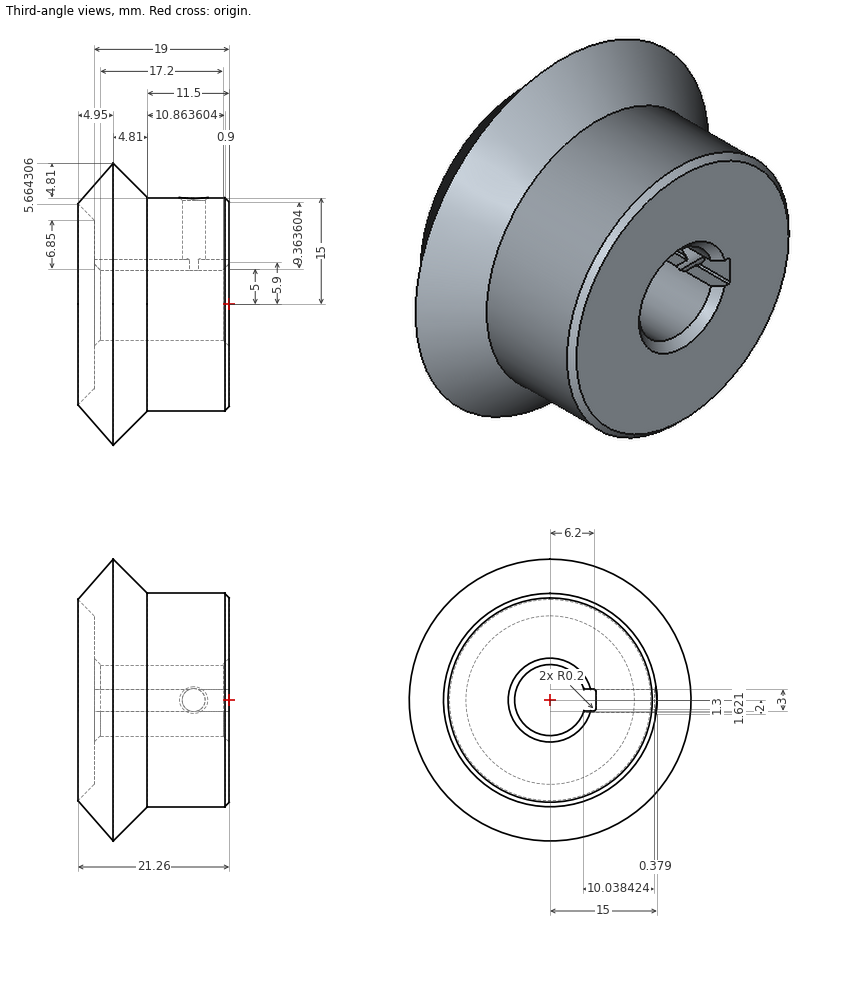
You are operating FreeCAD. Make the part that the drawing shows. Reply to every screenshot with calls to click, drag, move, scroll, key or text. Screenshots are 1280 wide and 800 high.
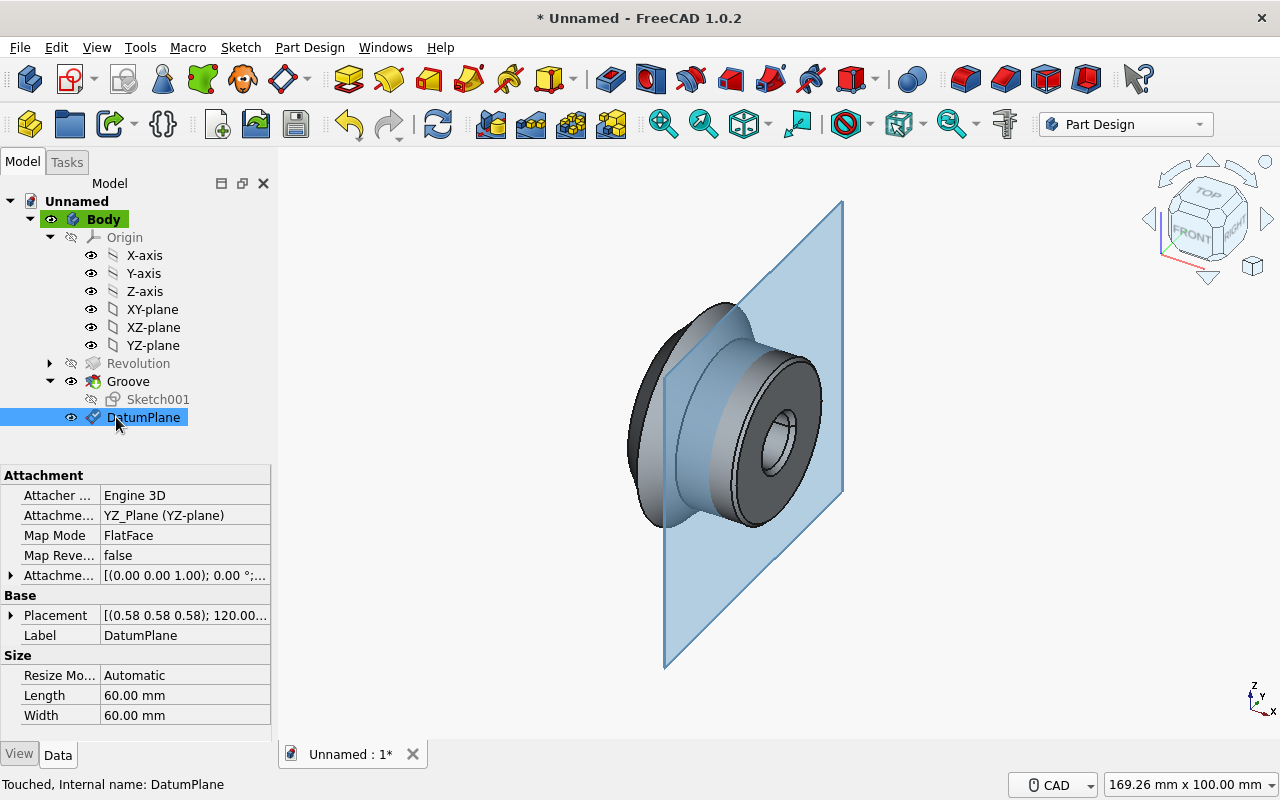
click(70, 80)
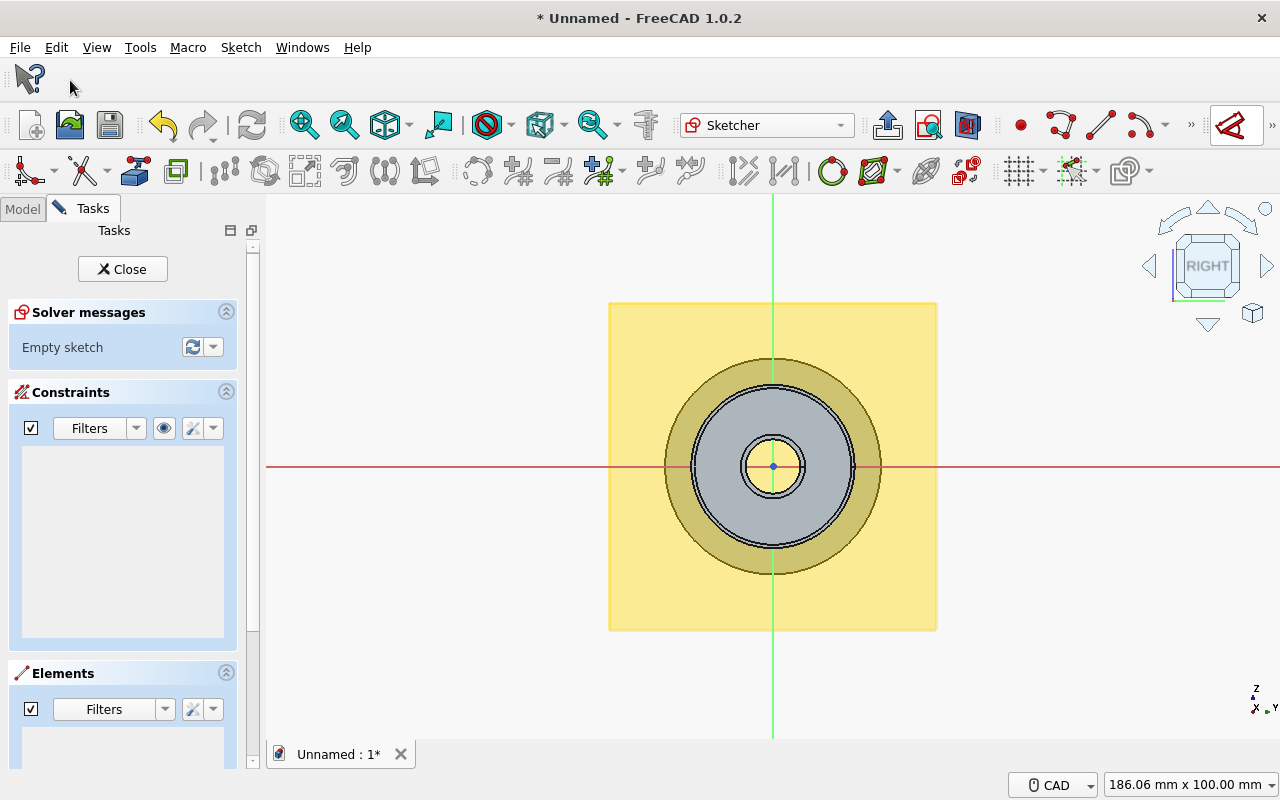
click(968, 126)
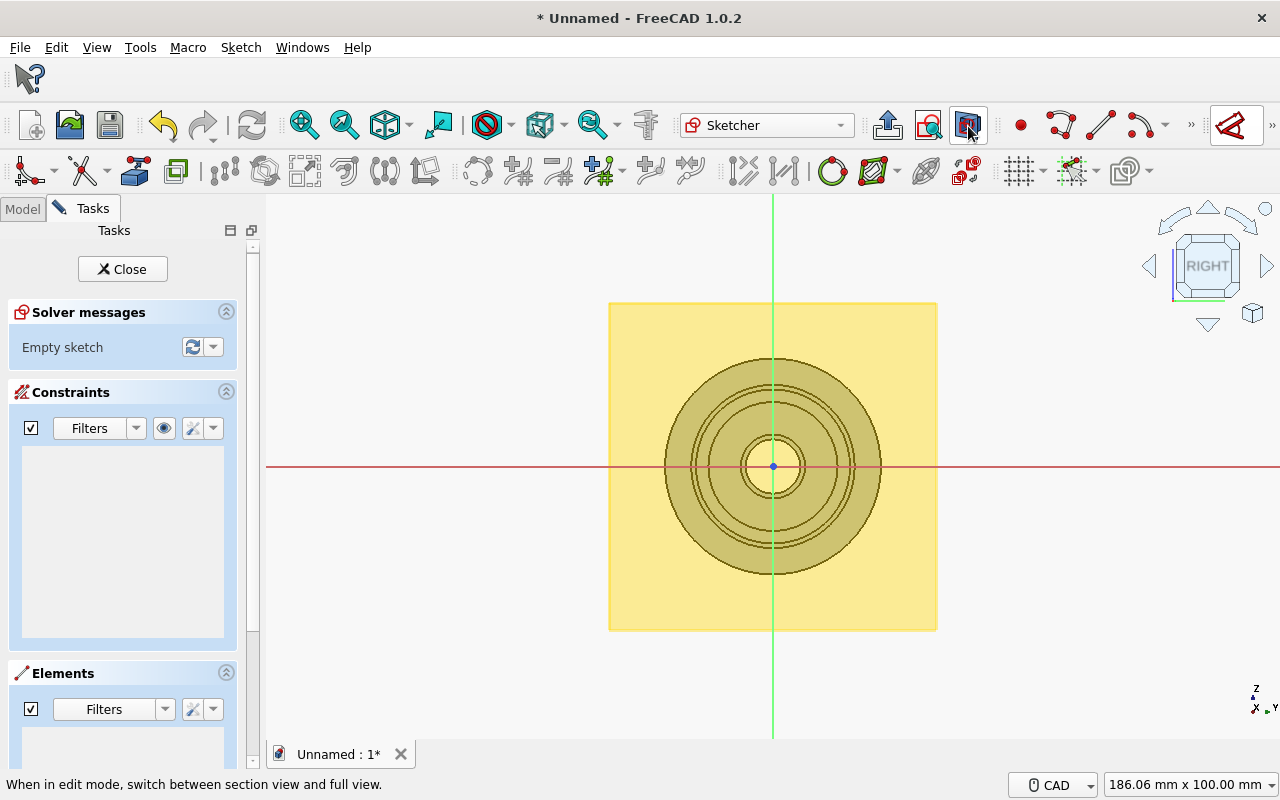
scroll(831, 473, up, 10)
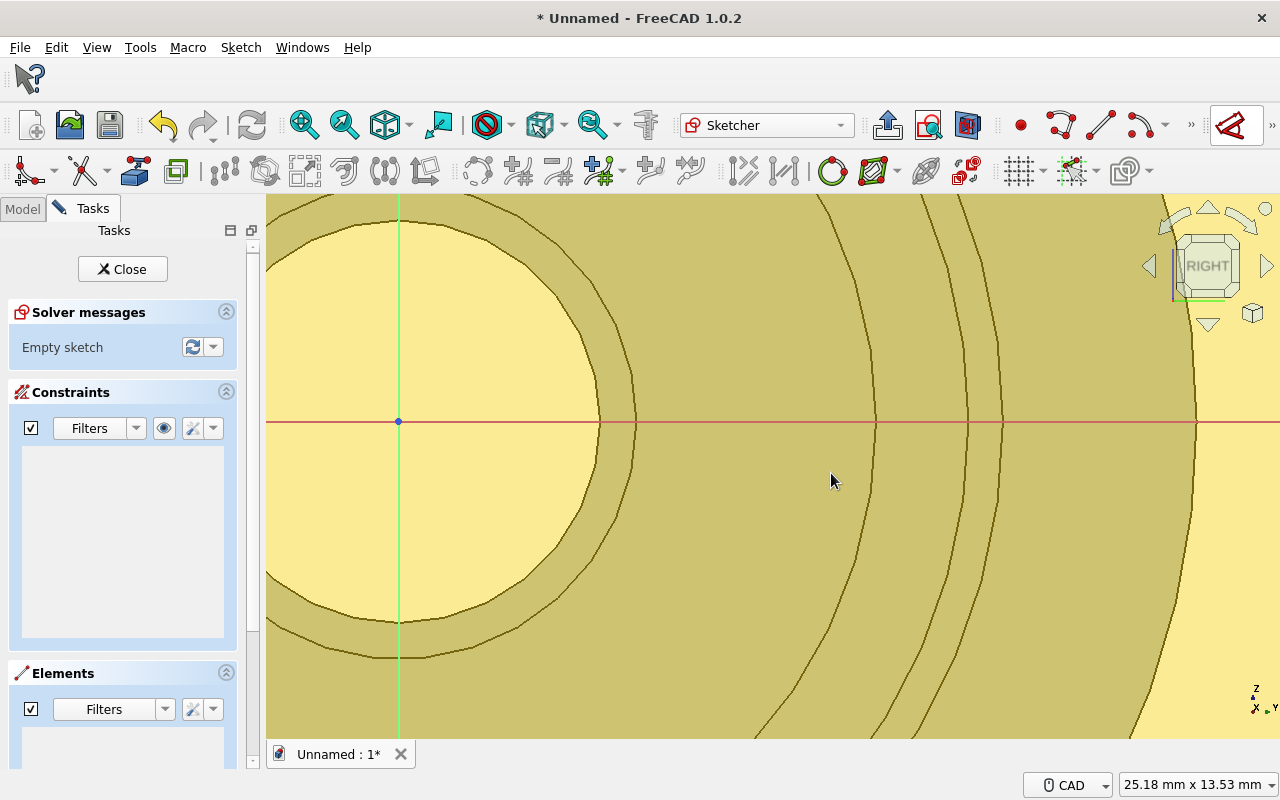
click(1062, 126)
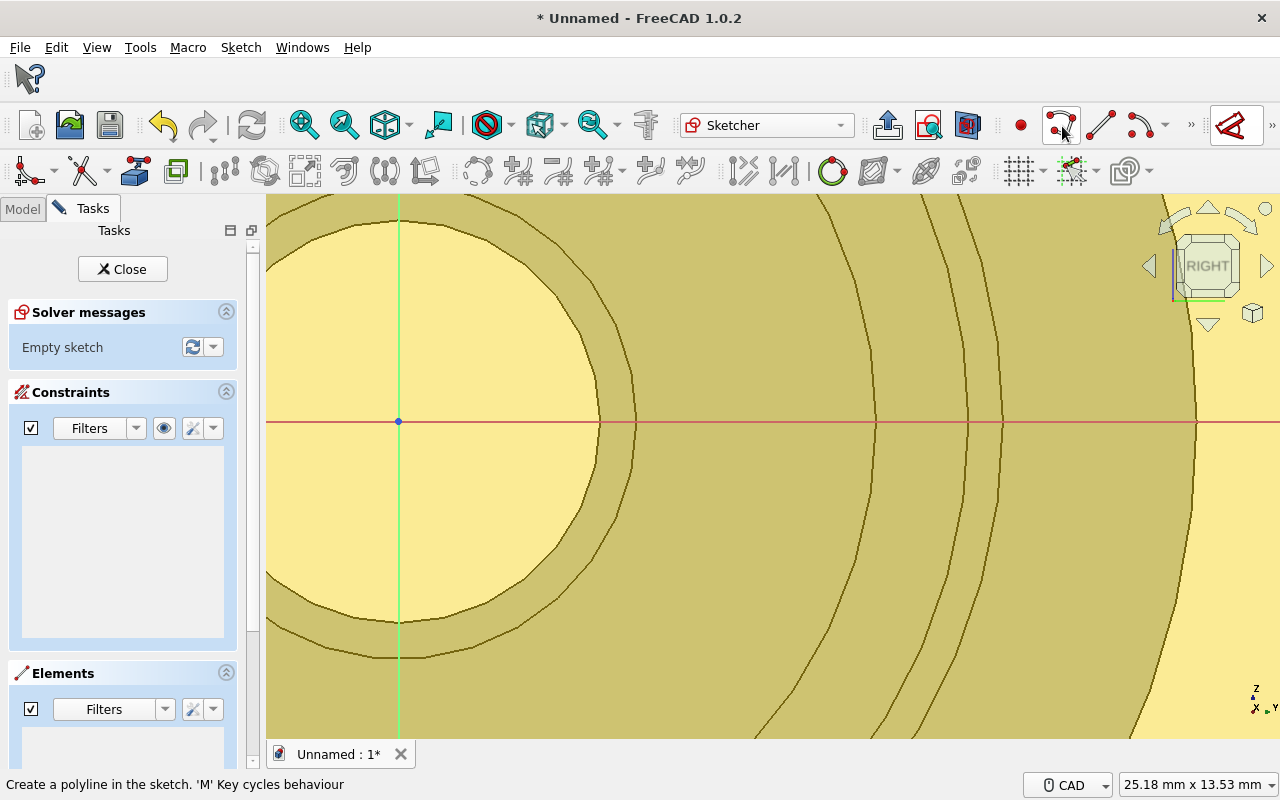
click(583, 422)
click(583, 487)
click(988, 487)
click(1003, 502)
click(1003, 431)
click(583, 422)
key(Escape)
key(Escape)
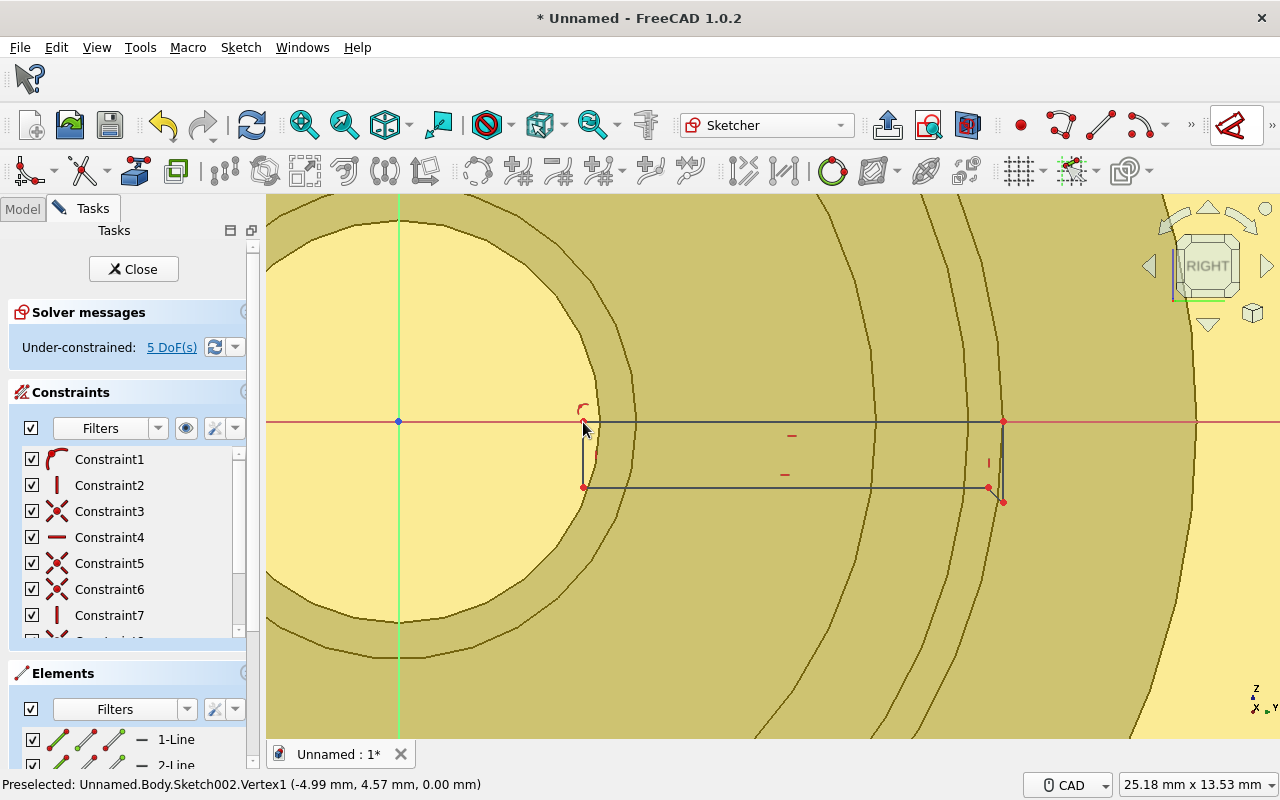
click(1003, 479)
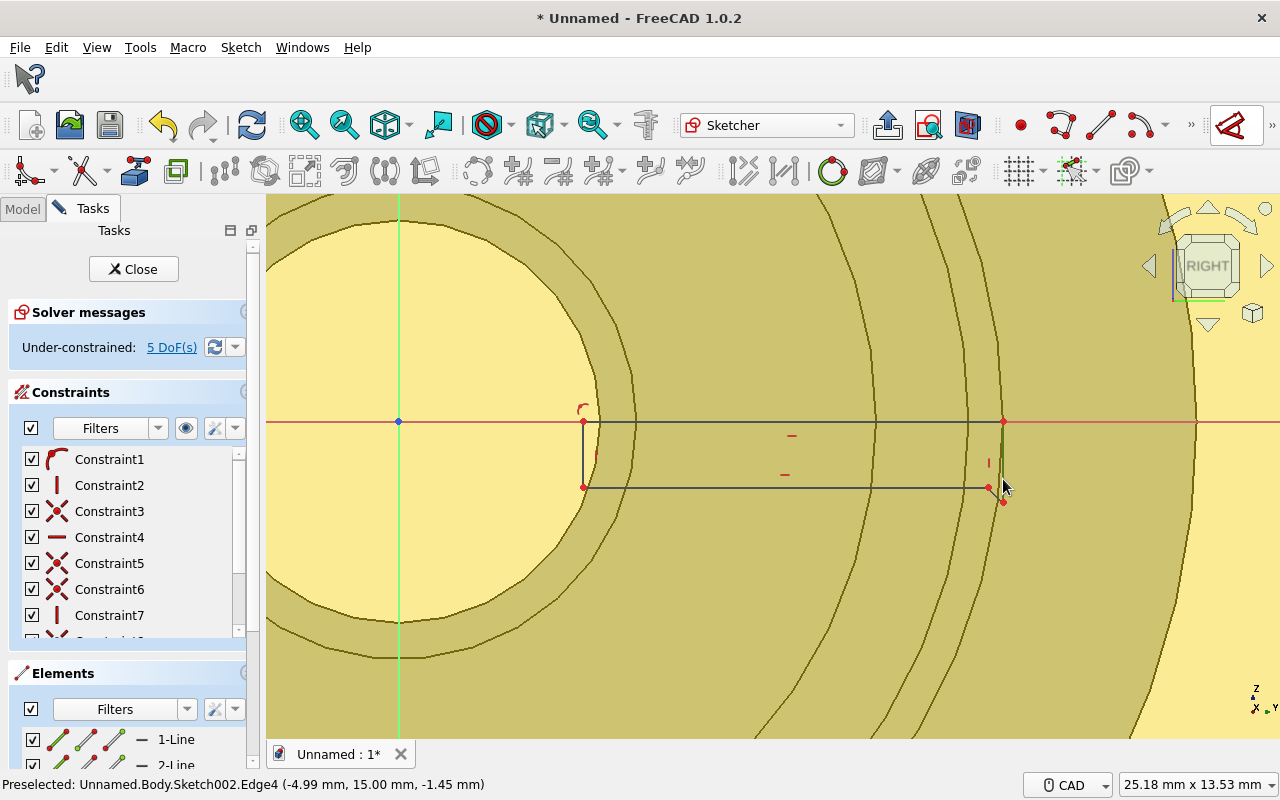
click(1258, 126)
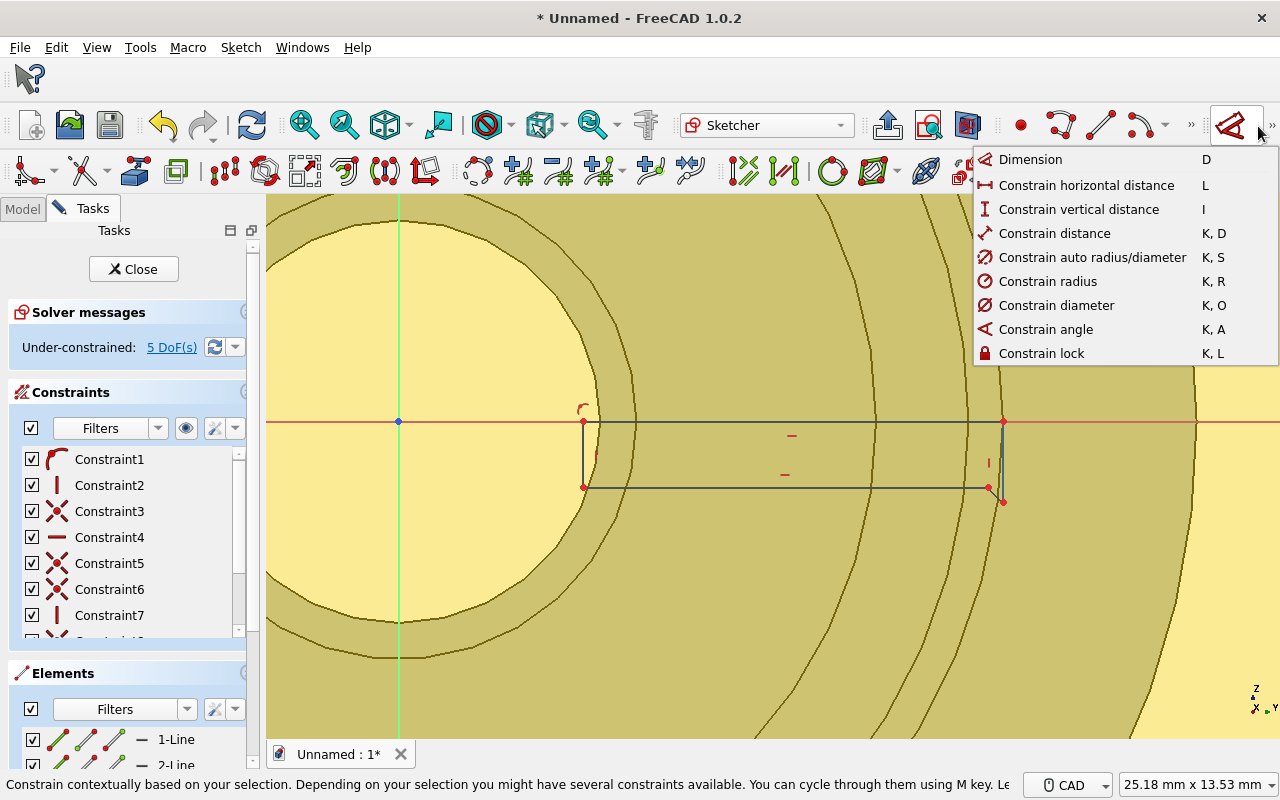
click(1126, 209)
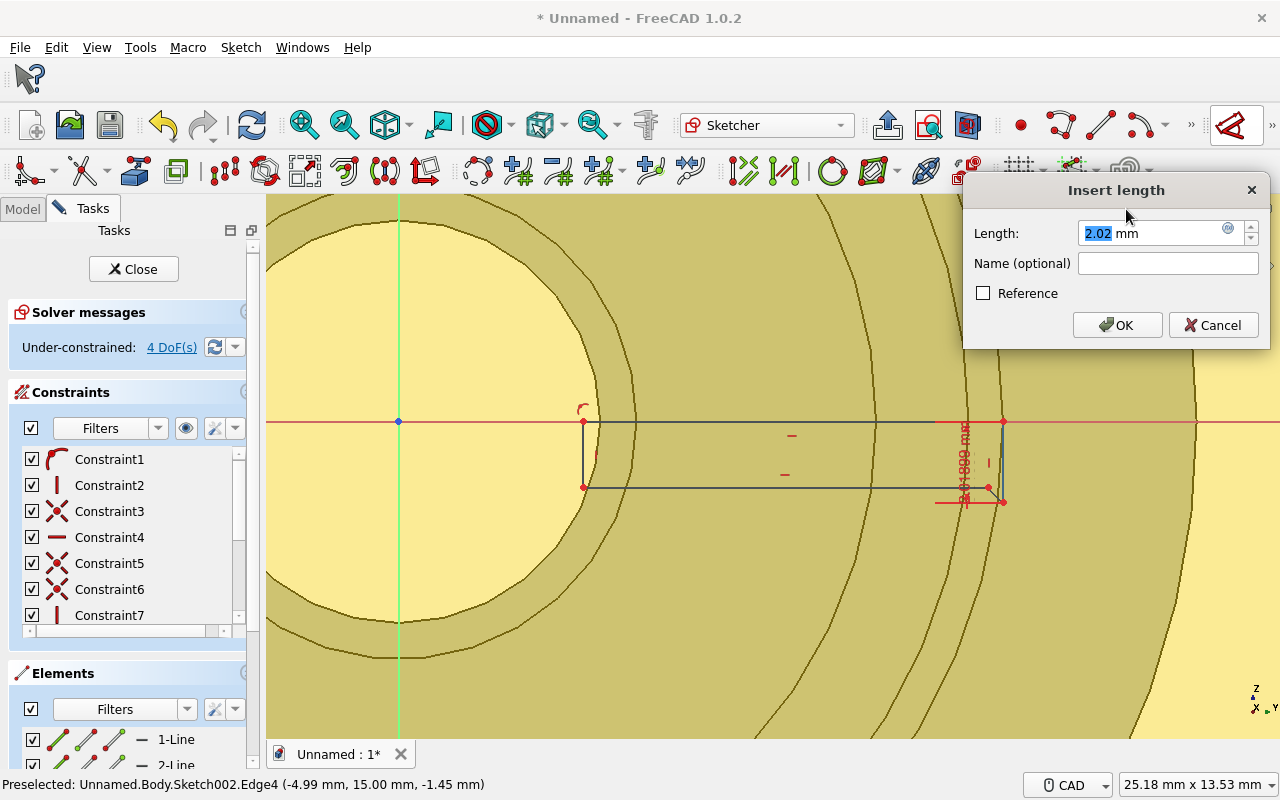
text(2)
key(Return)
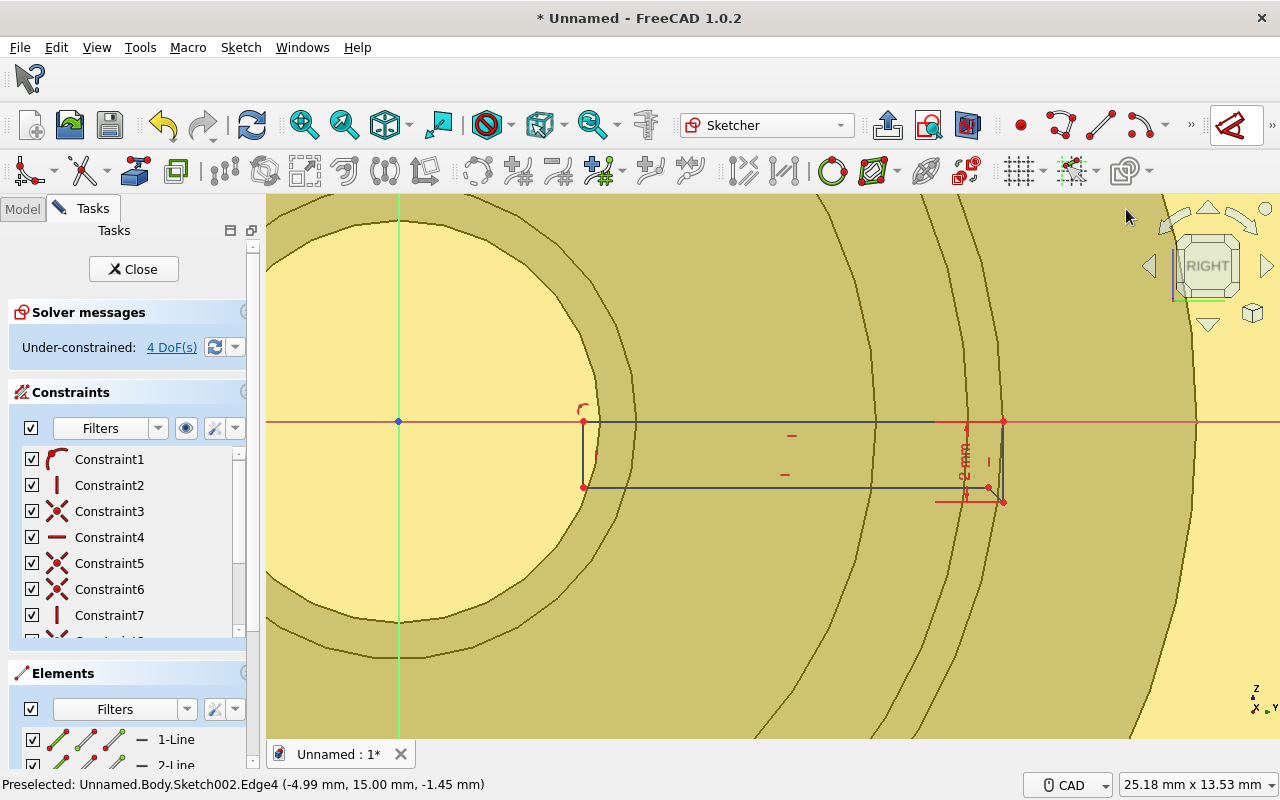
click(1003, 502)